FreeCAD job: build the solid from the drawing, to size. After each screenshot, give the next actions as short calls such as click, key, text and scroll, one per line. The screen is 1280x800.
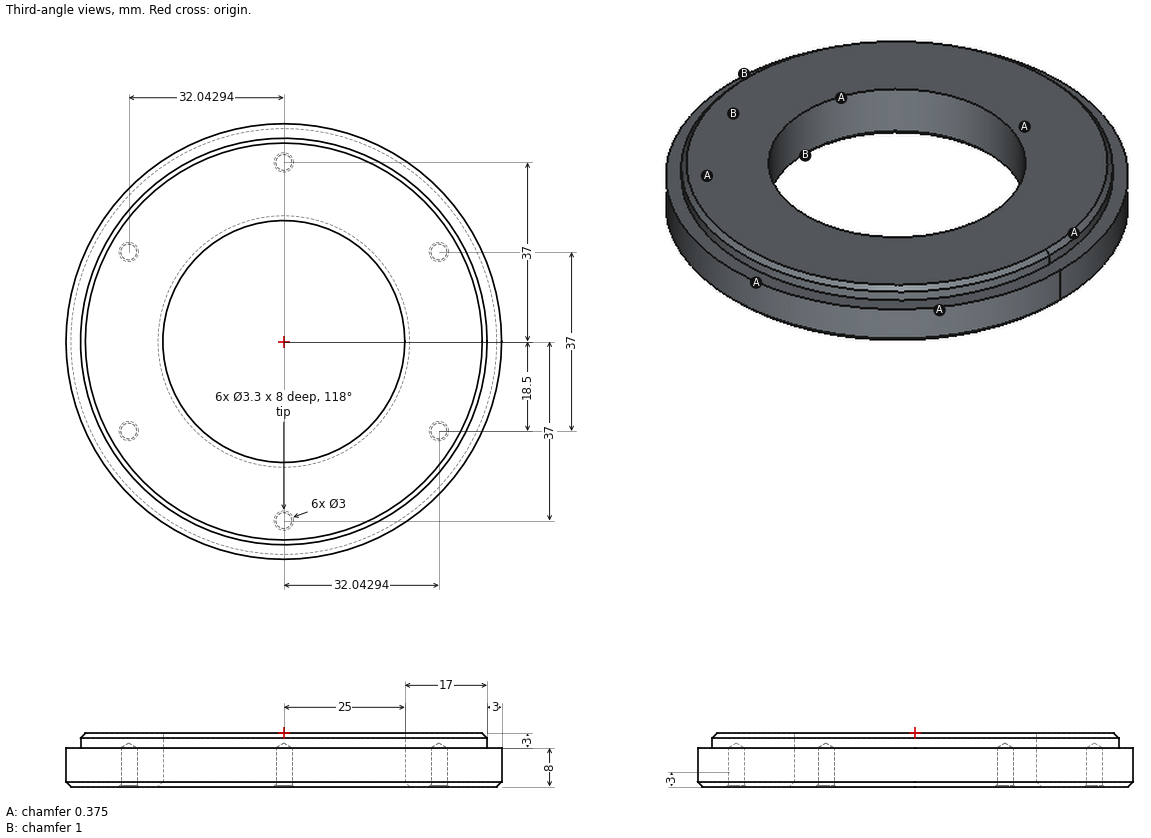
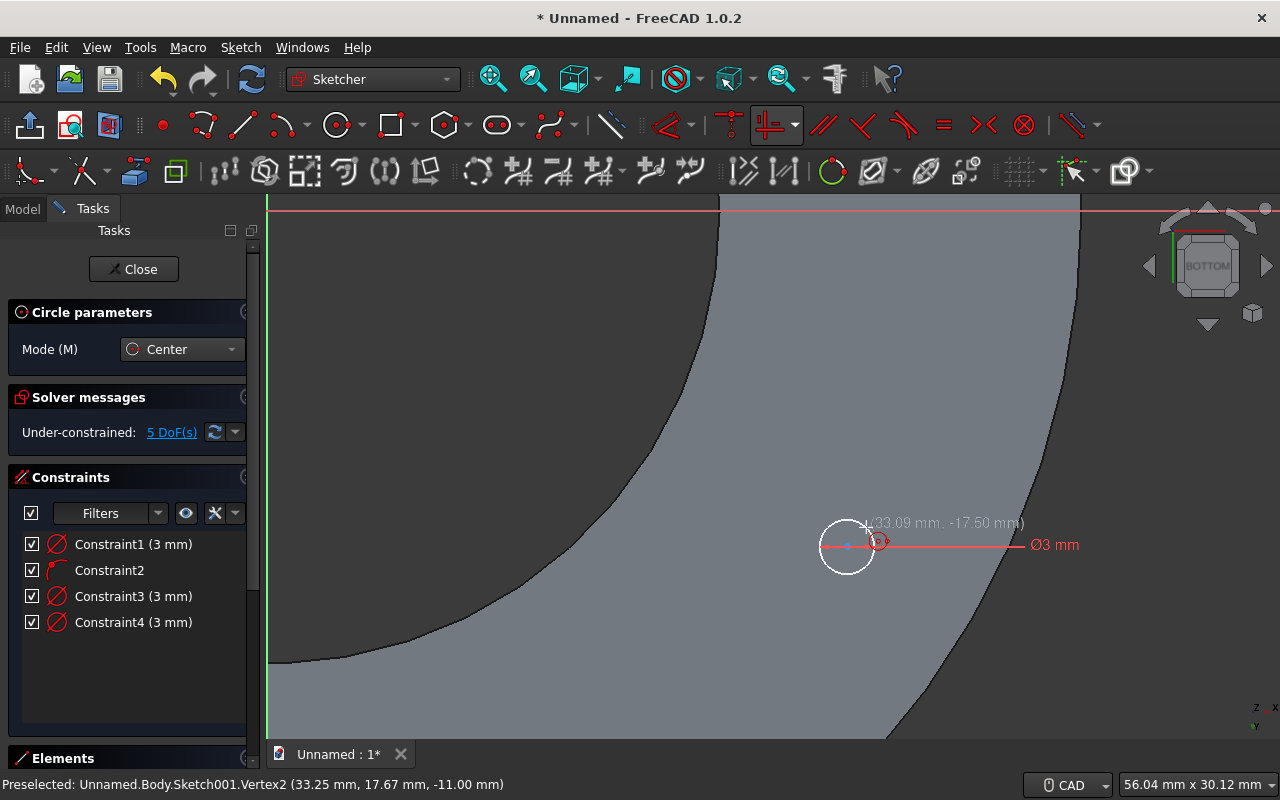
scroll(848, 550, down, 7)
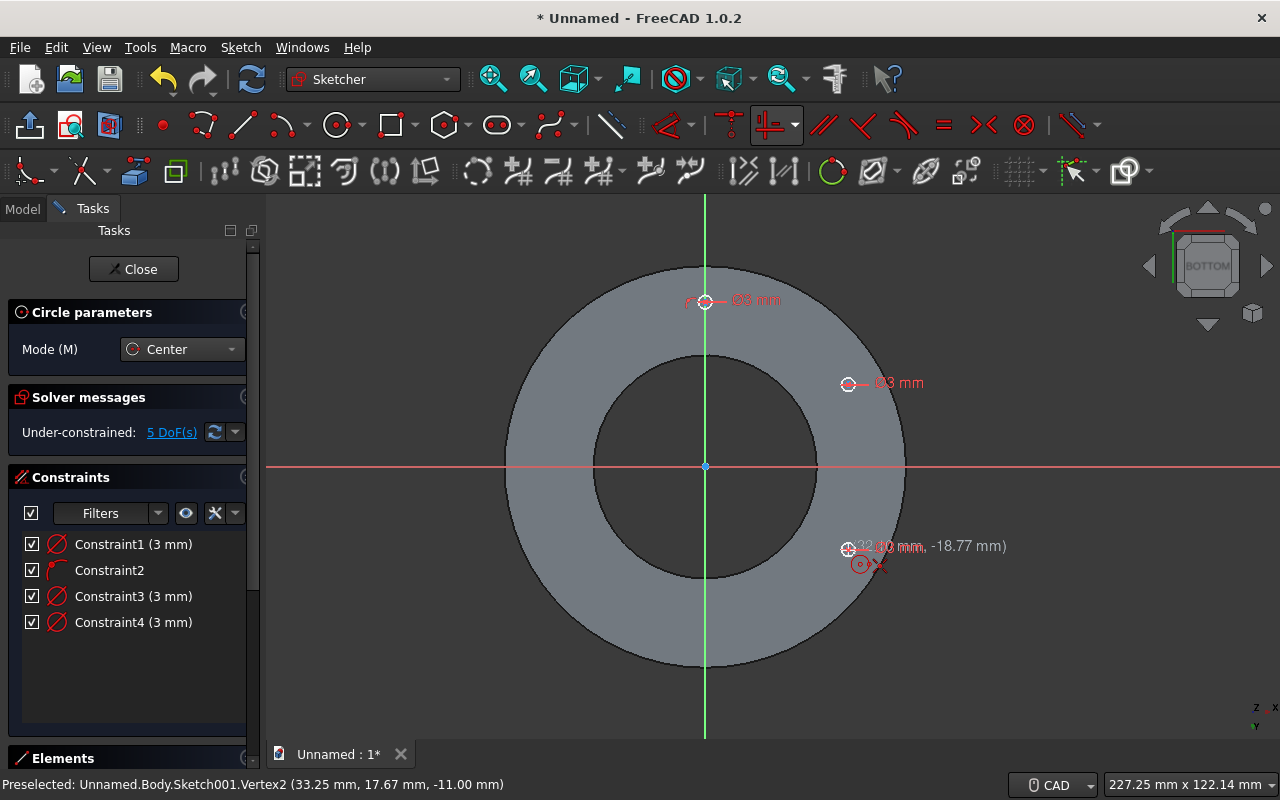
scroll(705, 632, up, 7)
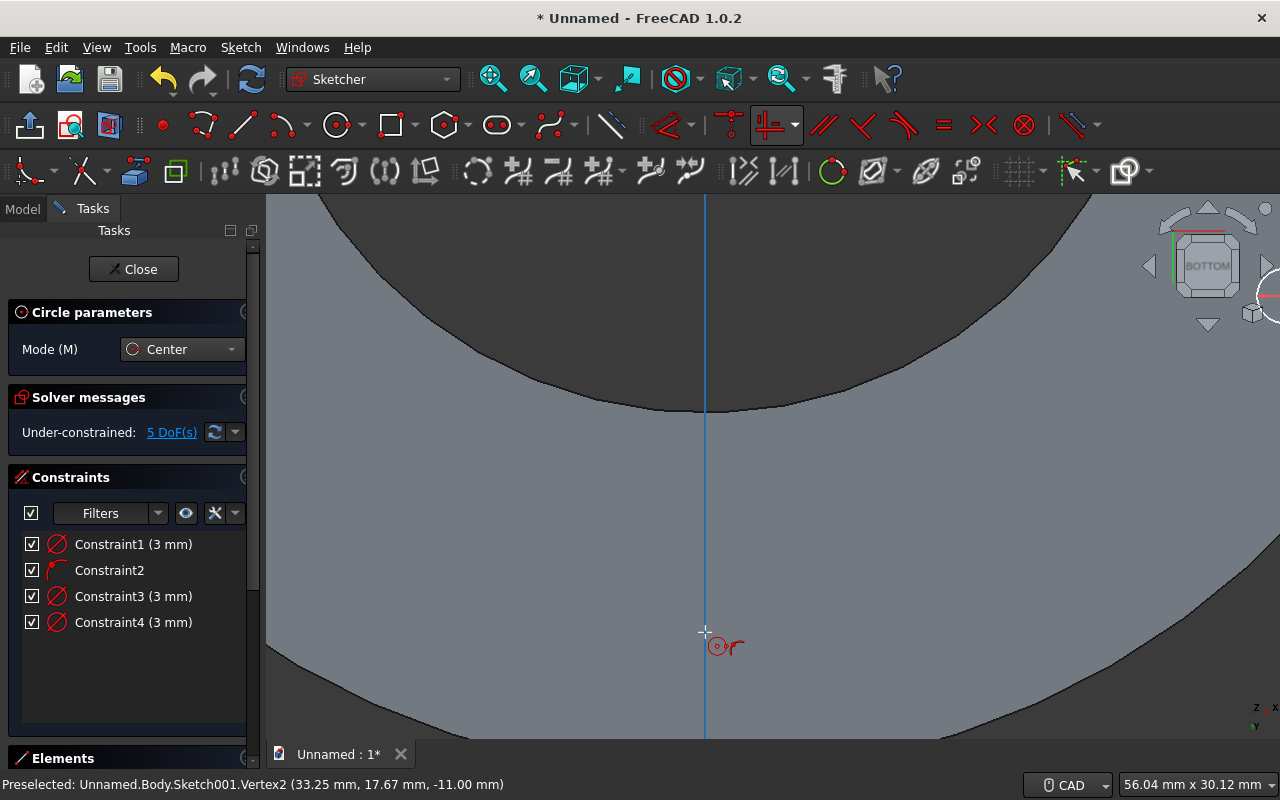
click(705, 630)
move(724, 611)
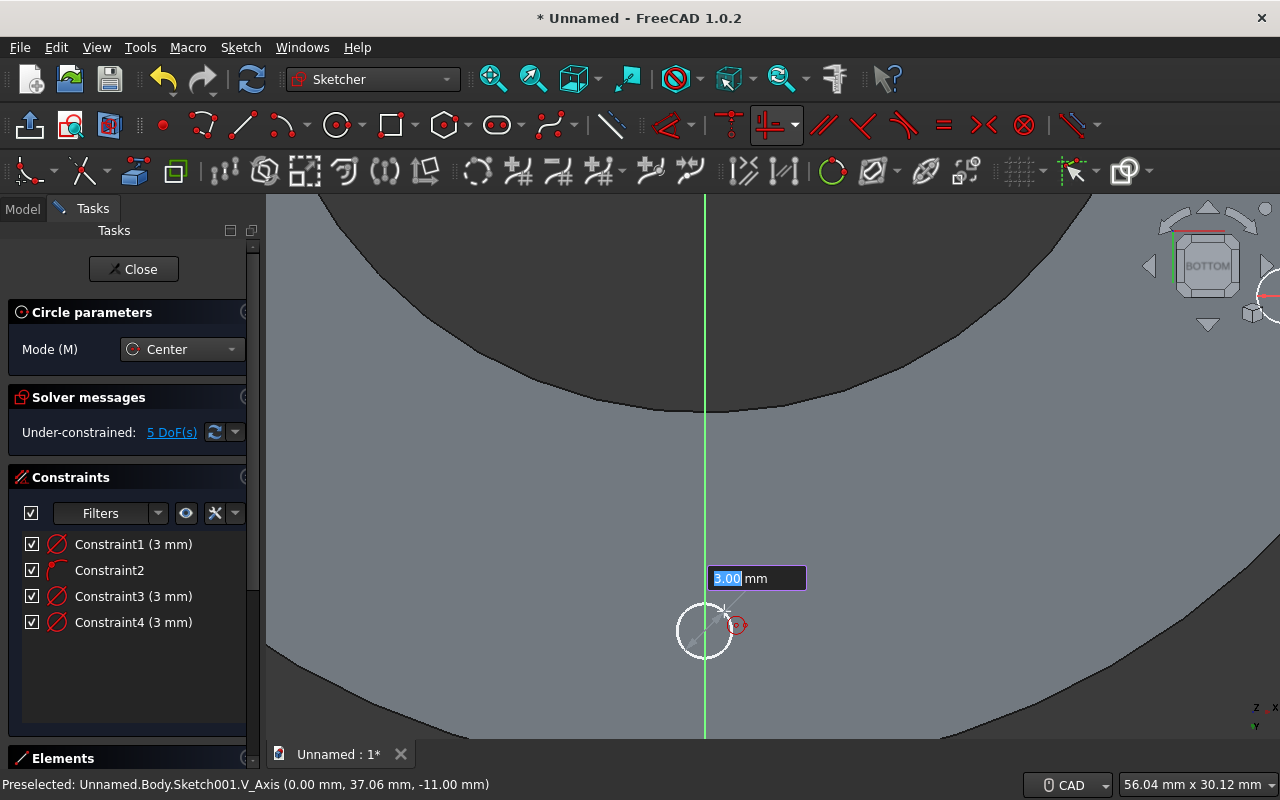
text(3)
key(Return)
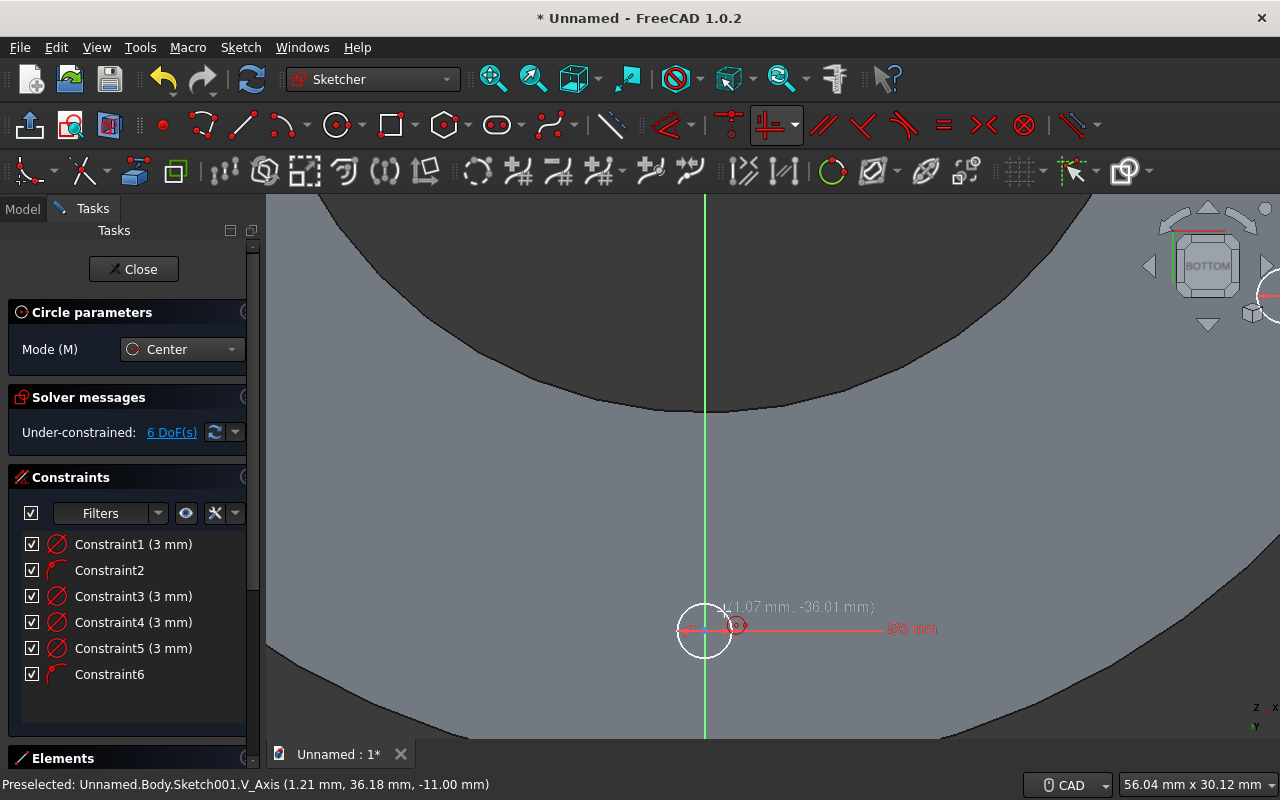
scroll(704, 632, down, 7)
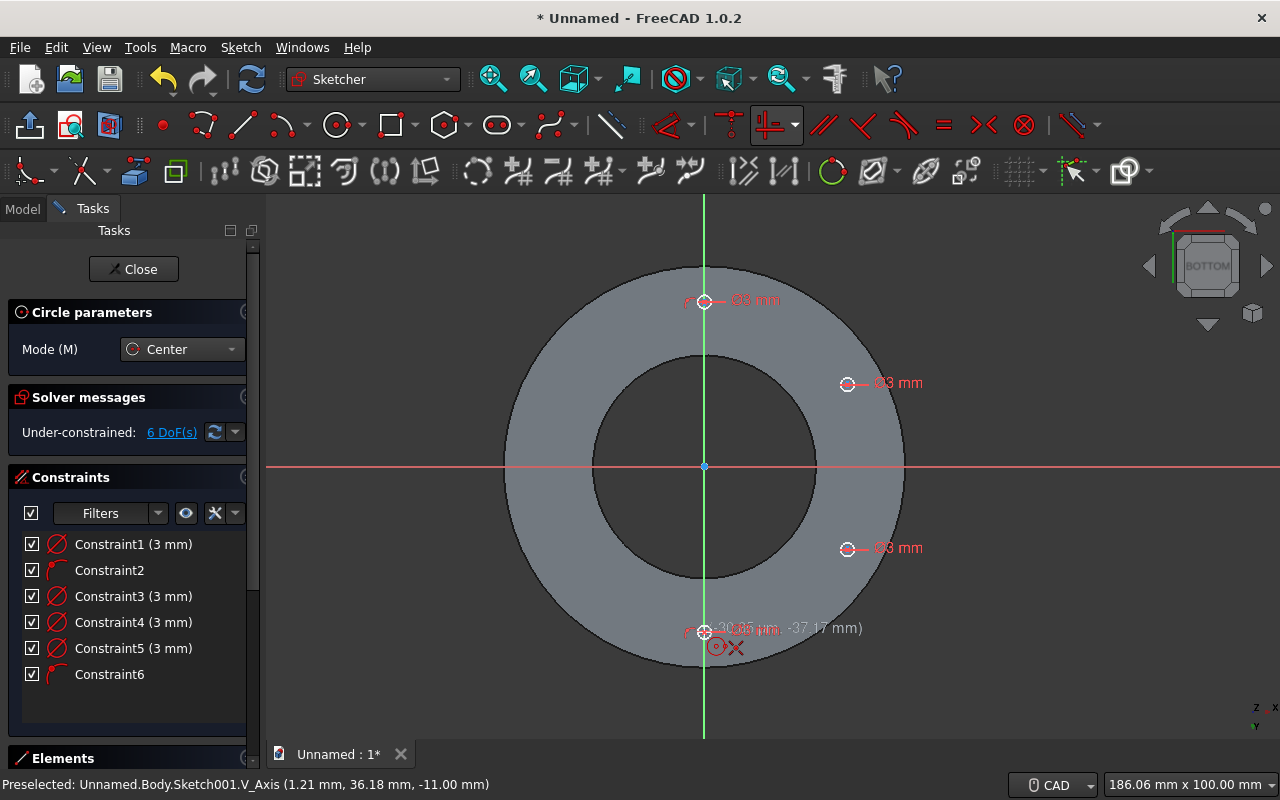
scroll(561, 550, up, 7)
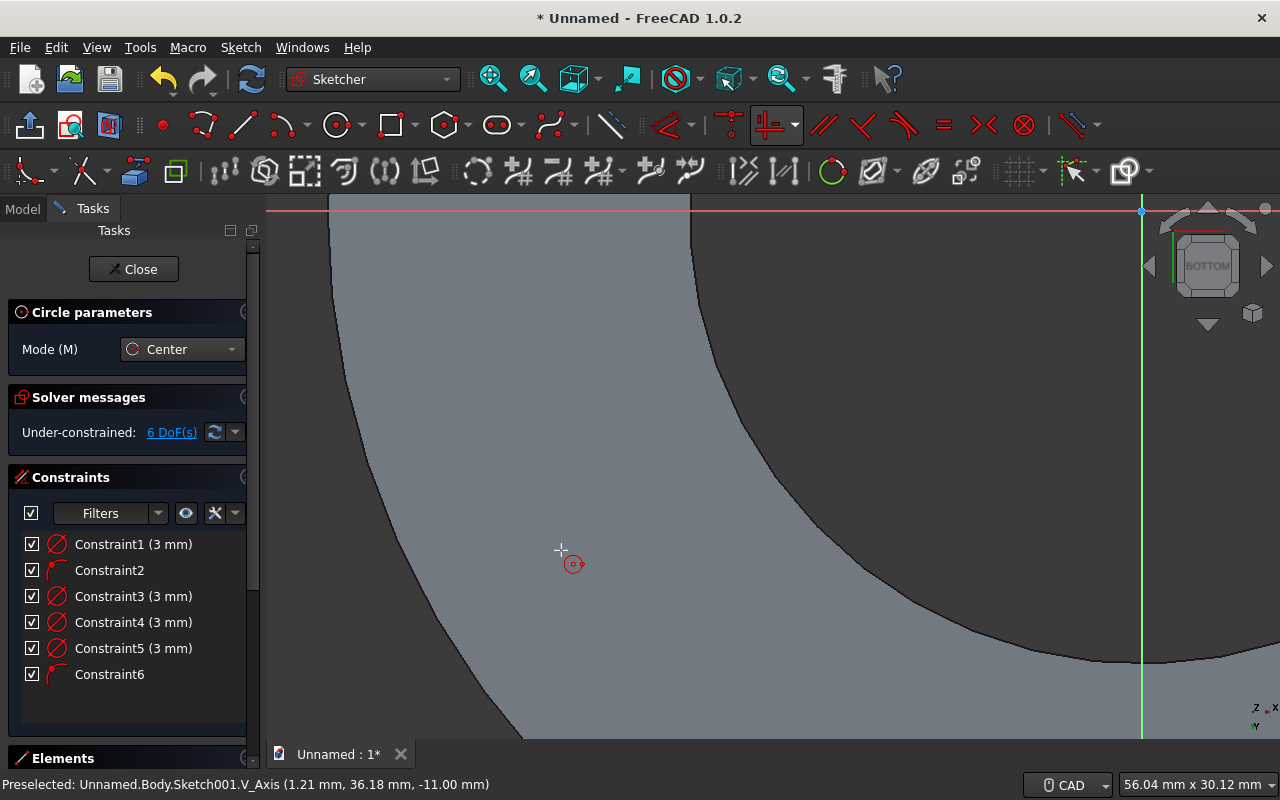
click(562, 546)
move(581, 527)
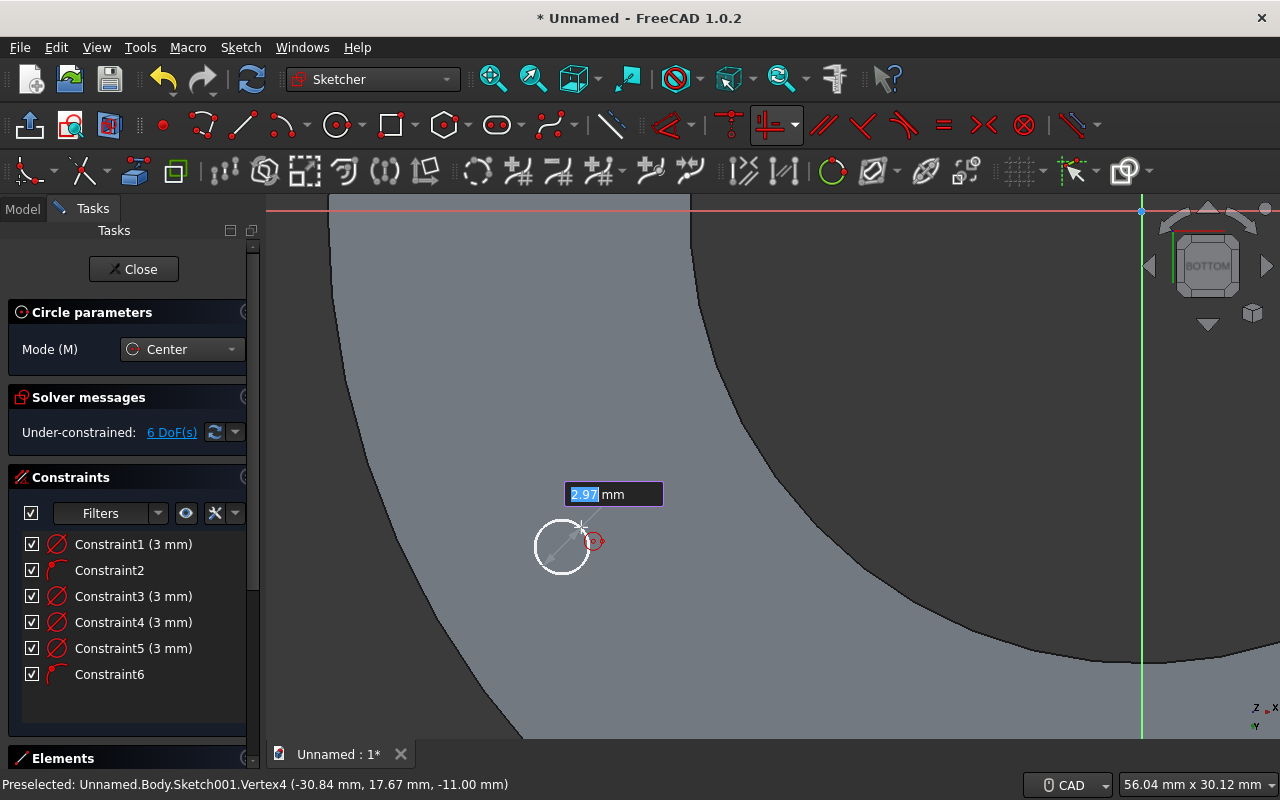
text(3)
key(Return)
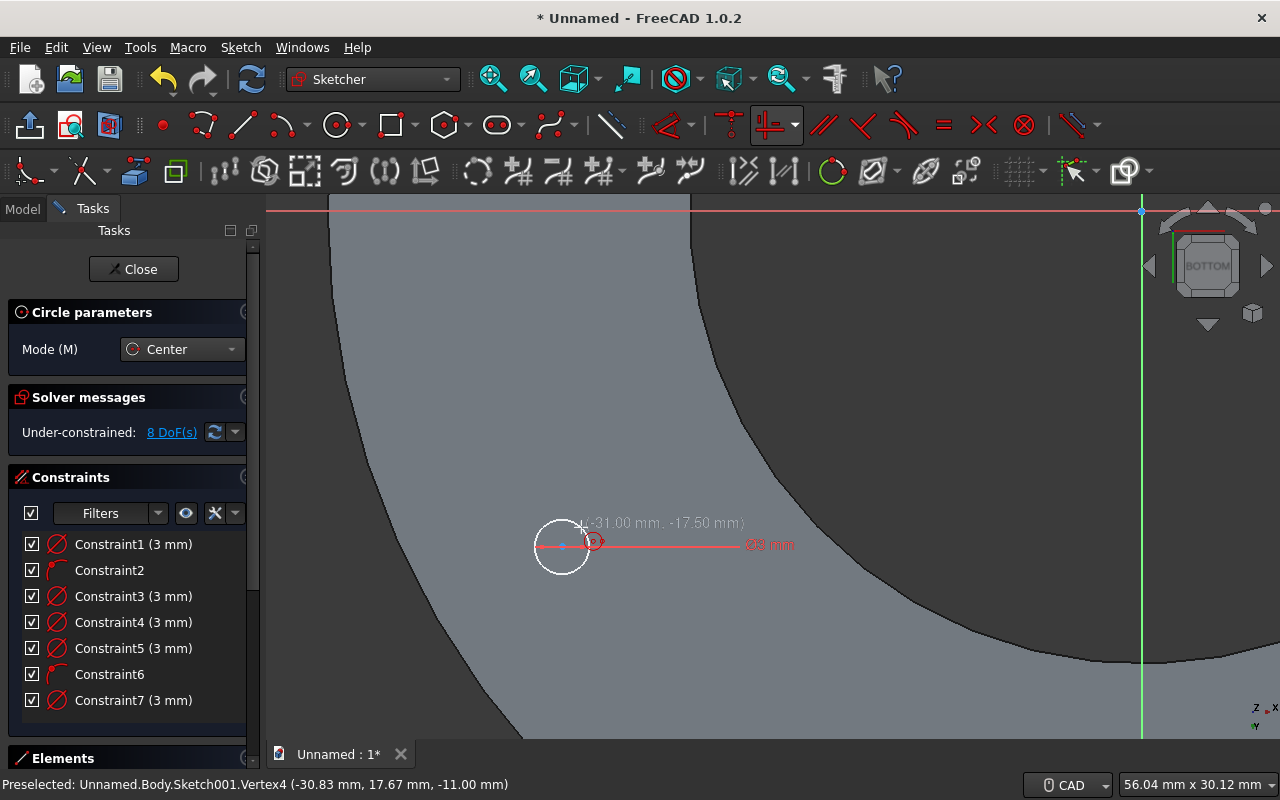
scroll(561, 550, down, 7)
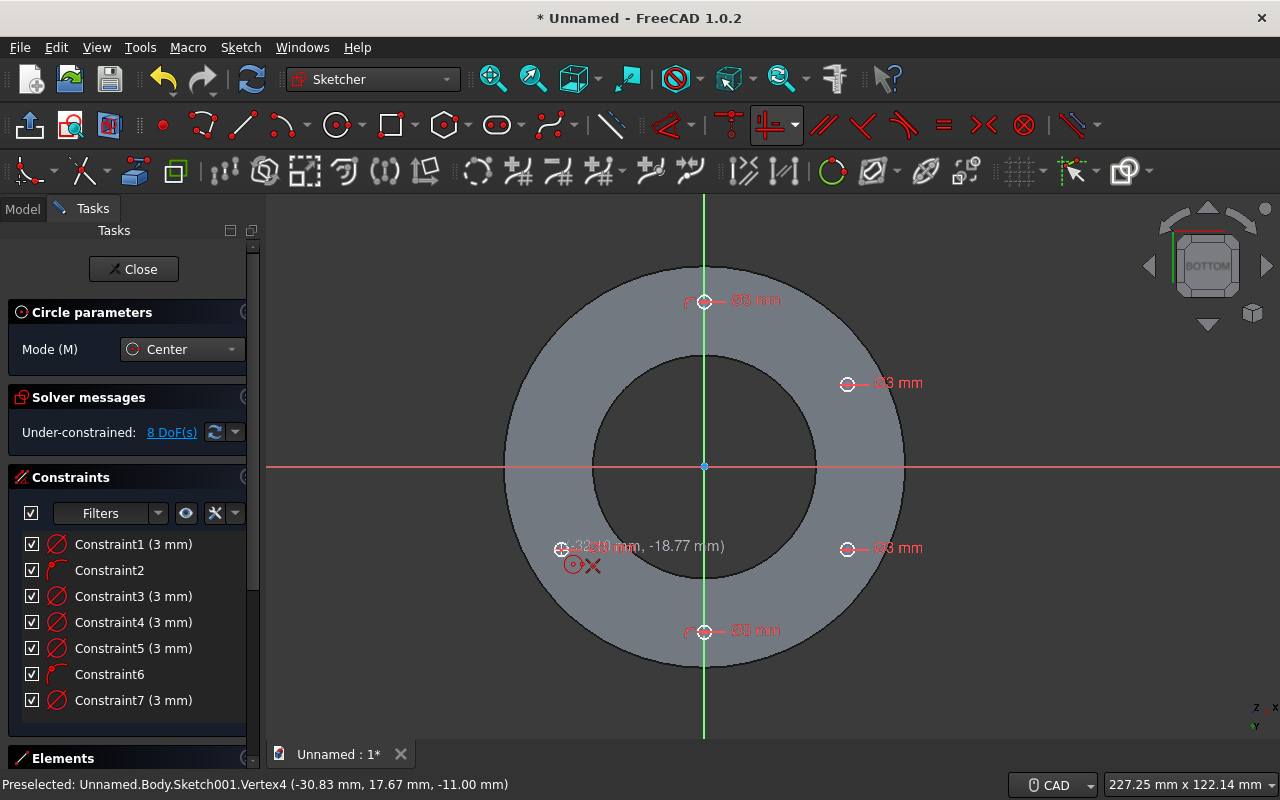
scroll(561, 384, up, 7)